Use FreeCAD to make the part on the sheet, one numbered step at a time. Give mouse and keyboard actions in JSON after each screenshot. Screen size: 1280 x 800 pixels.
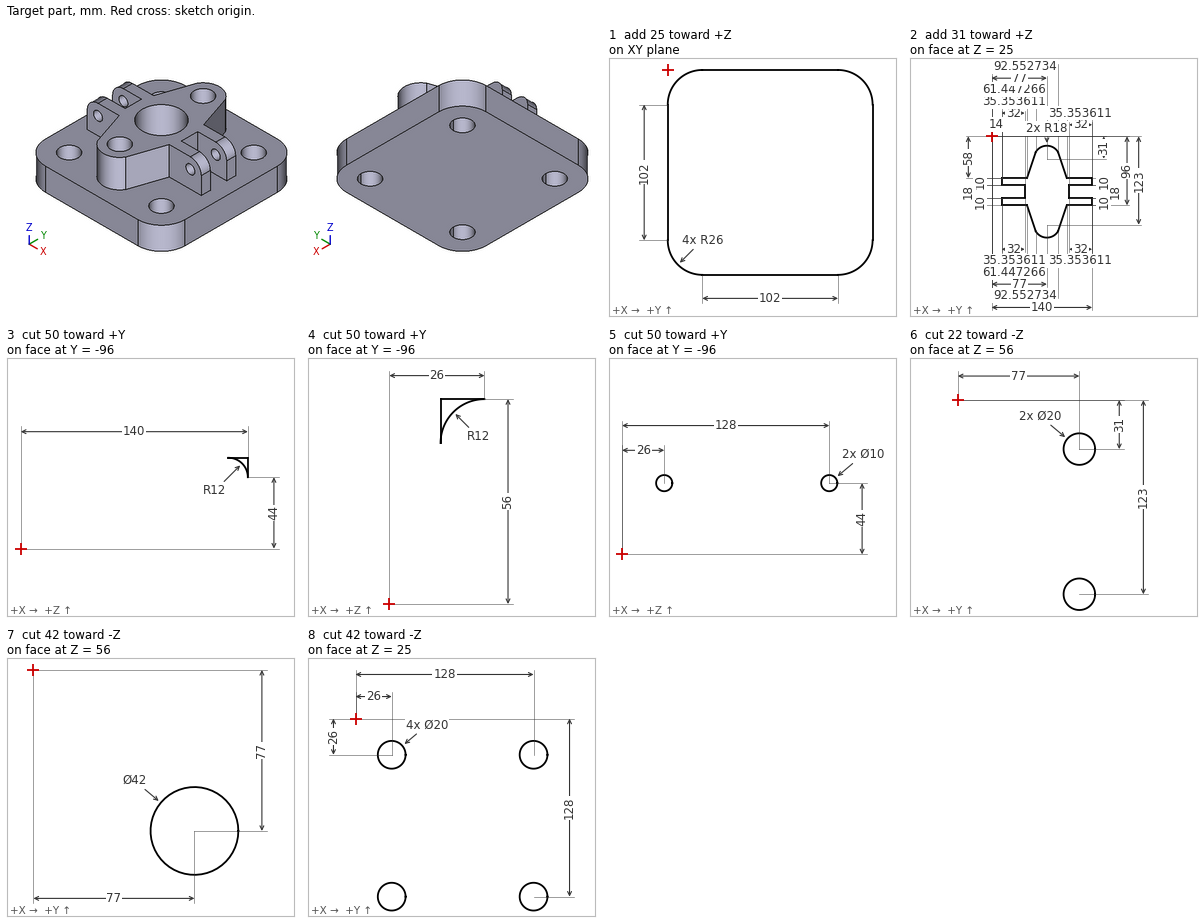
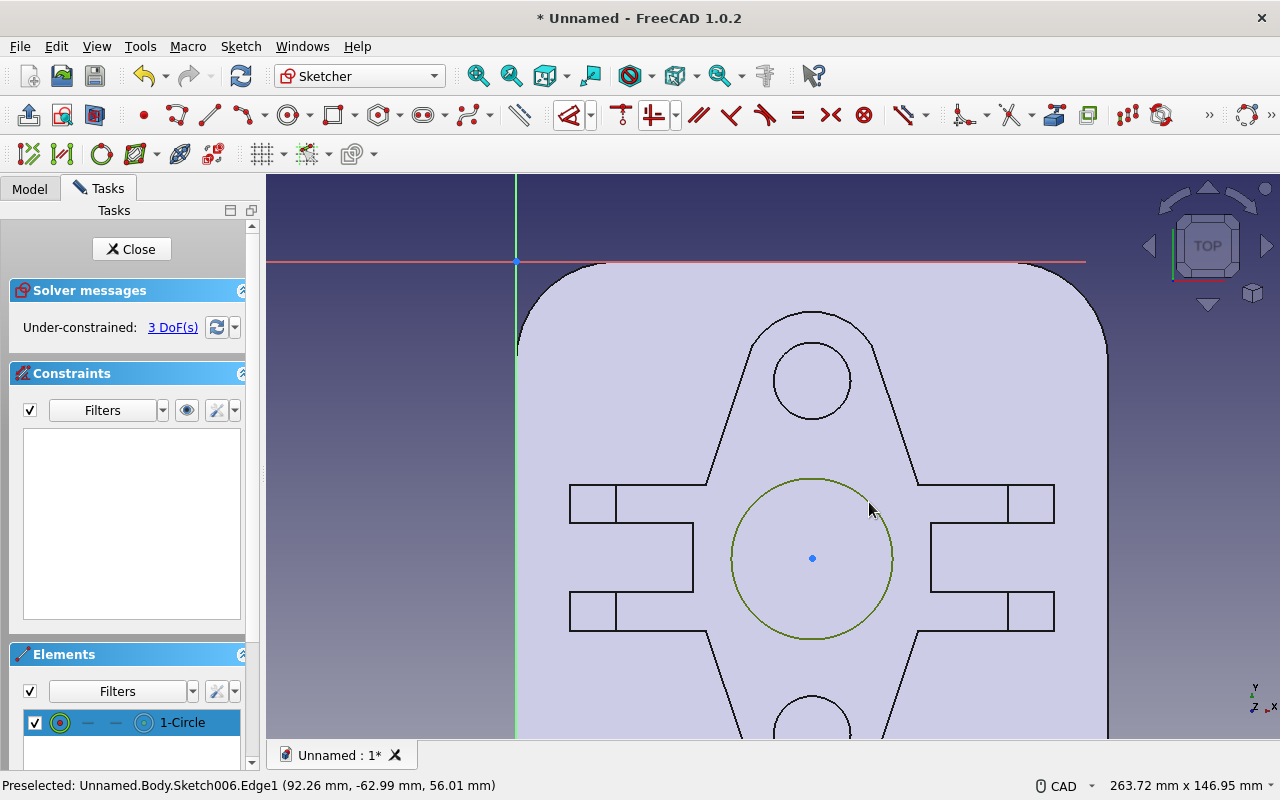
{"action": "key", "text": "k o"}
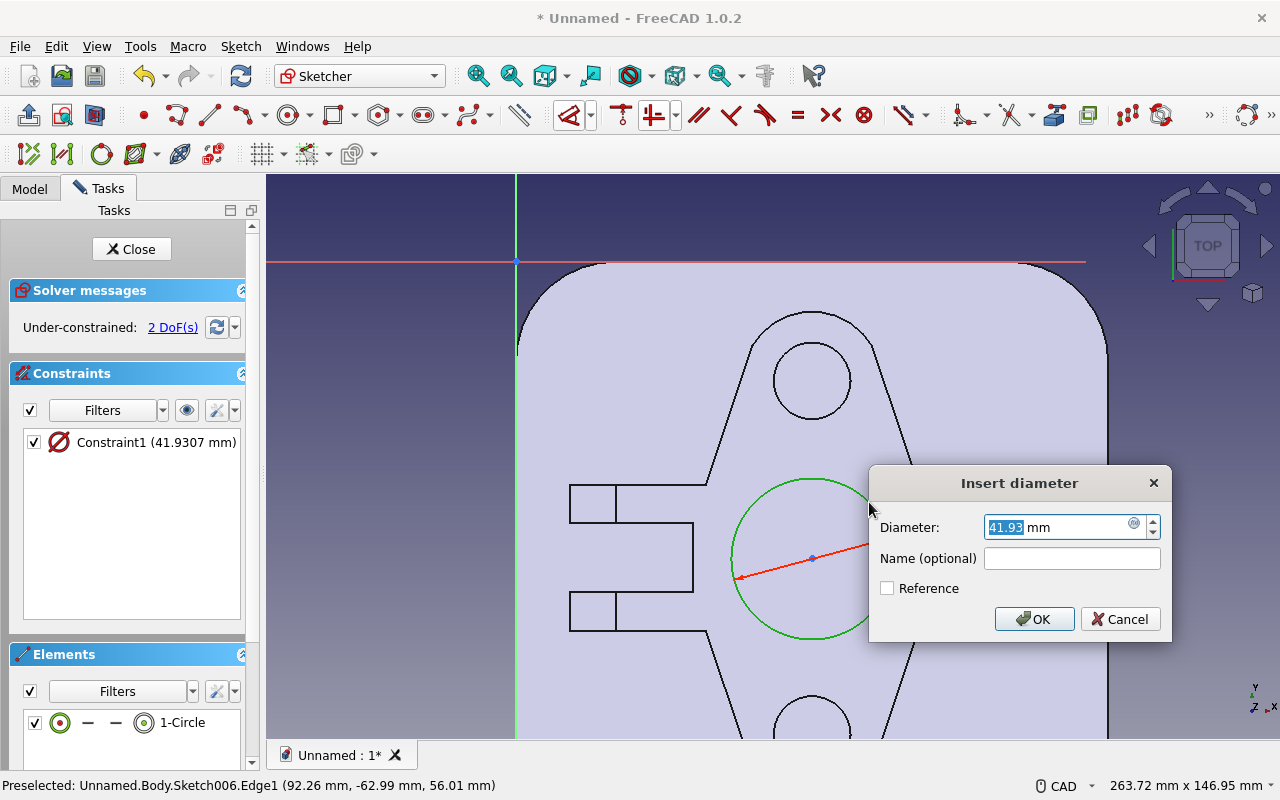
{"action": "type", "text": "42"}
{"action": "key", "text": "Return"}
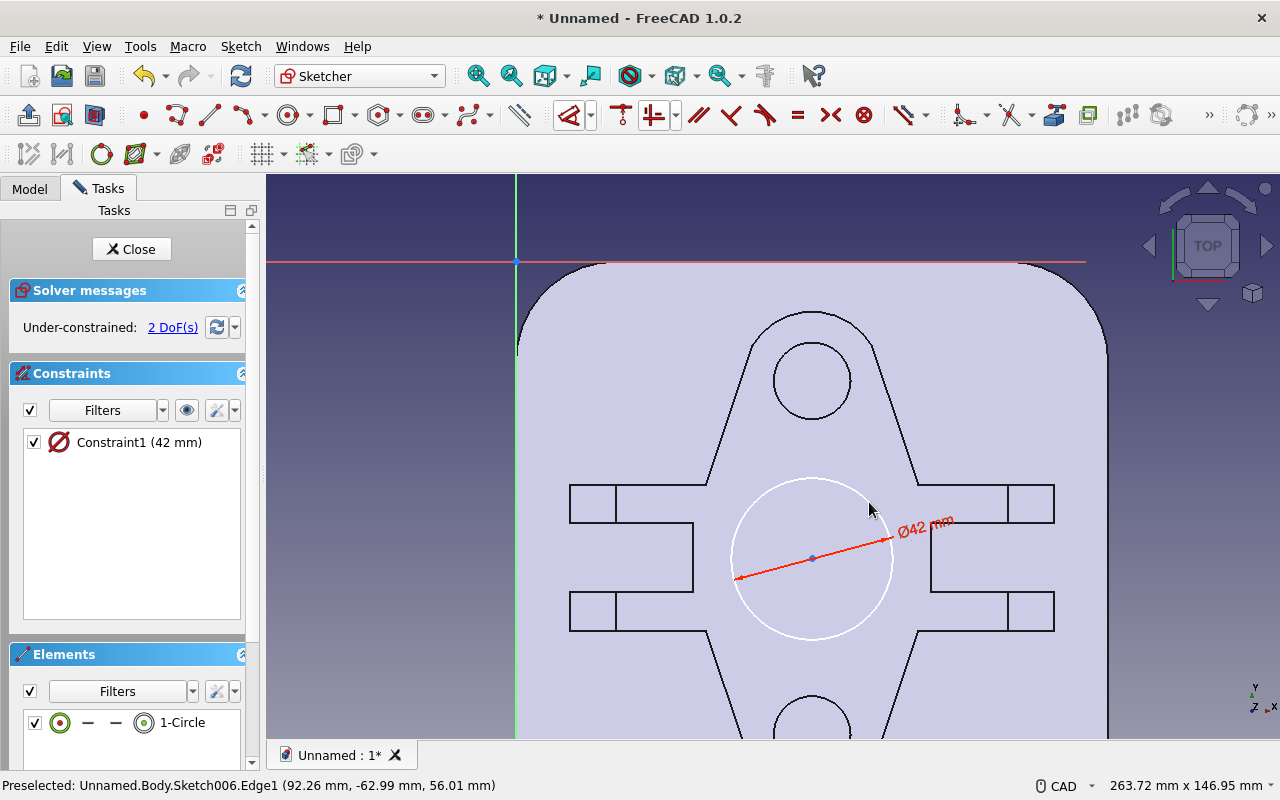
{"action": "left_click", "coordinate": [812, 559]}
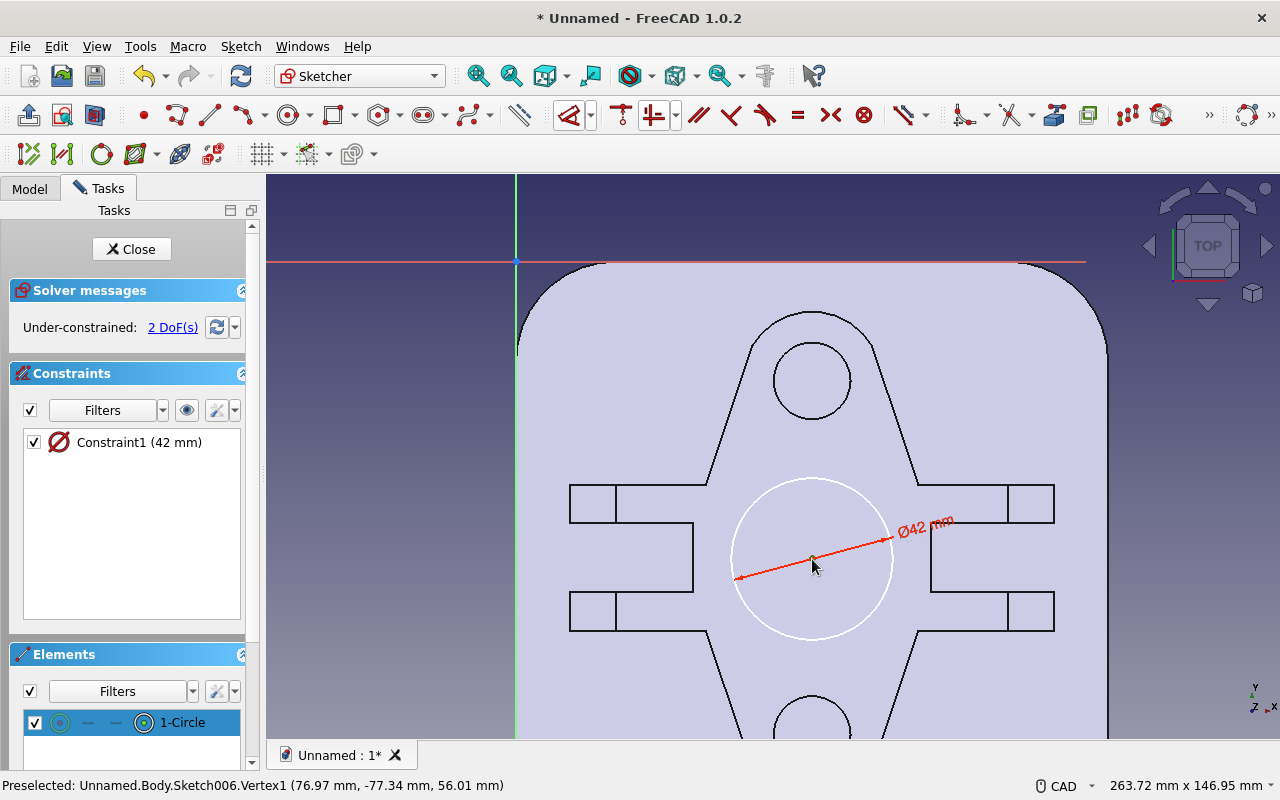
{"action": "left_click", "coordinate": [590, 116]}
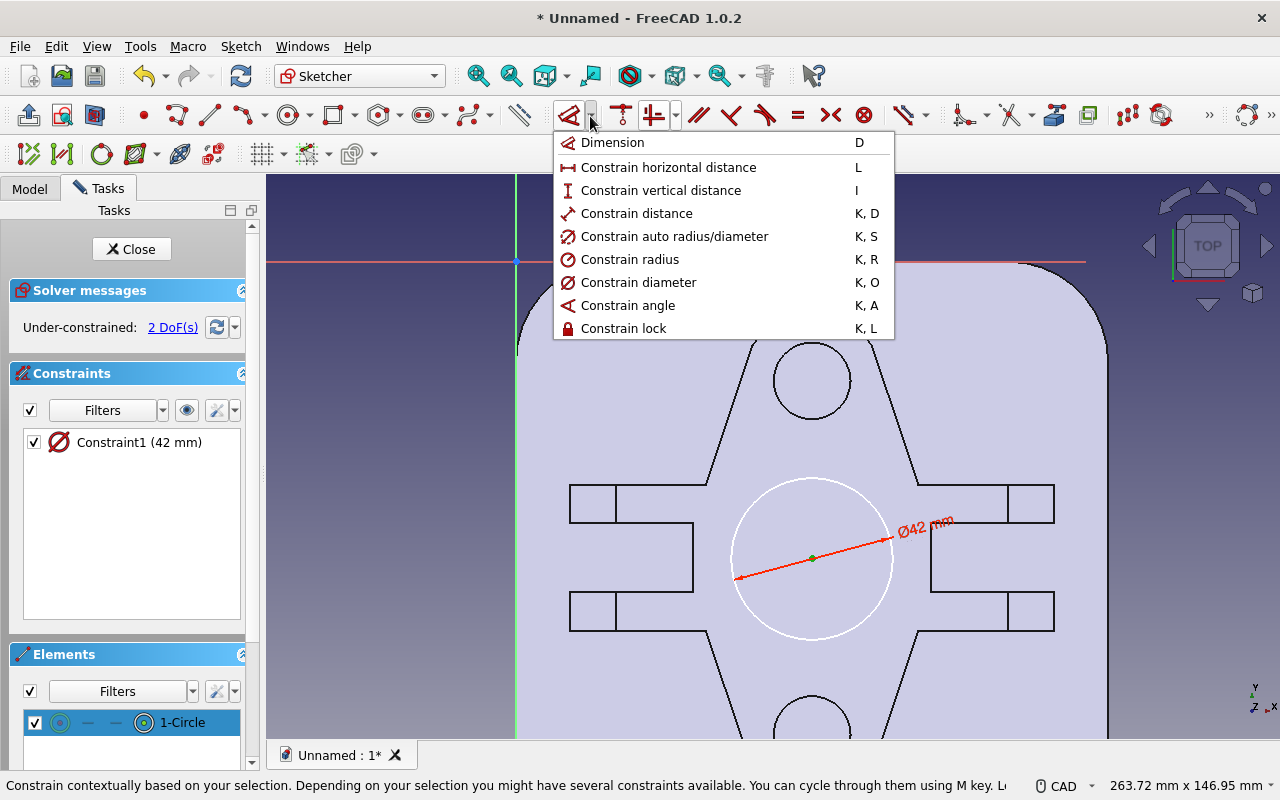
{"action": "left_click", "coordinate": [724, 168]}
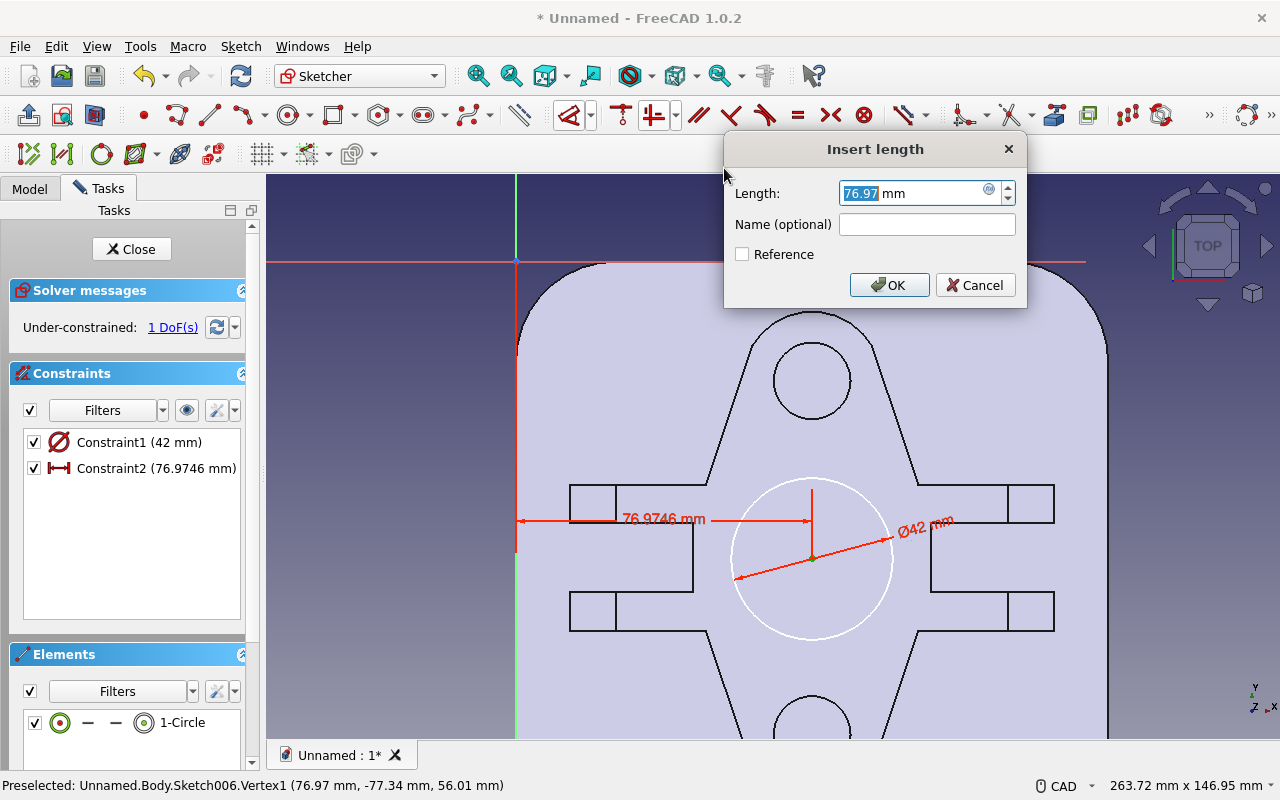
{"action": "type", "text": "77"}
{"action": "key", "text": "Return"}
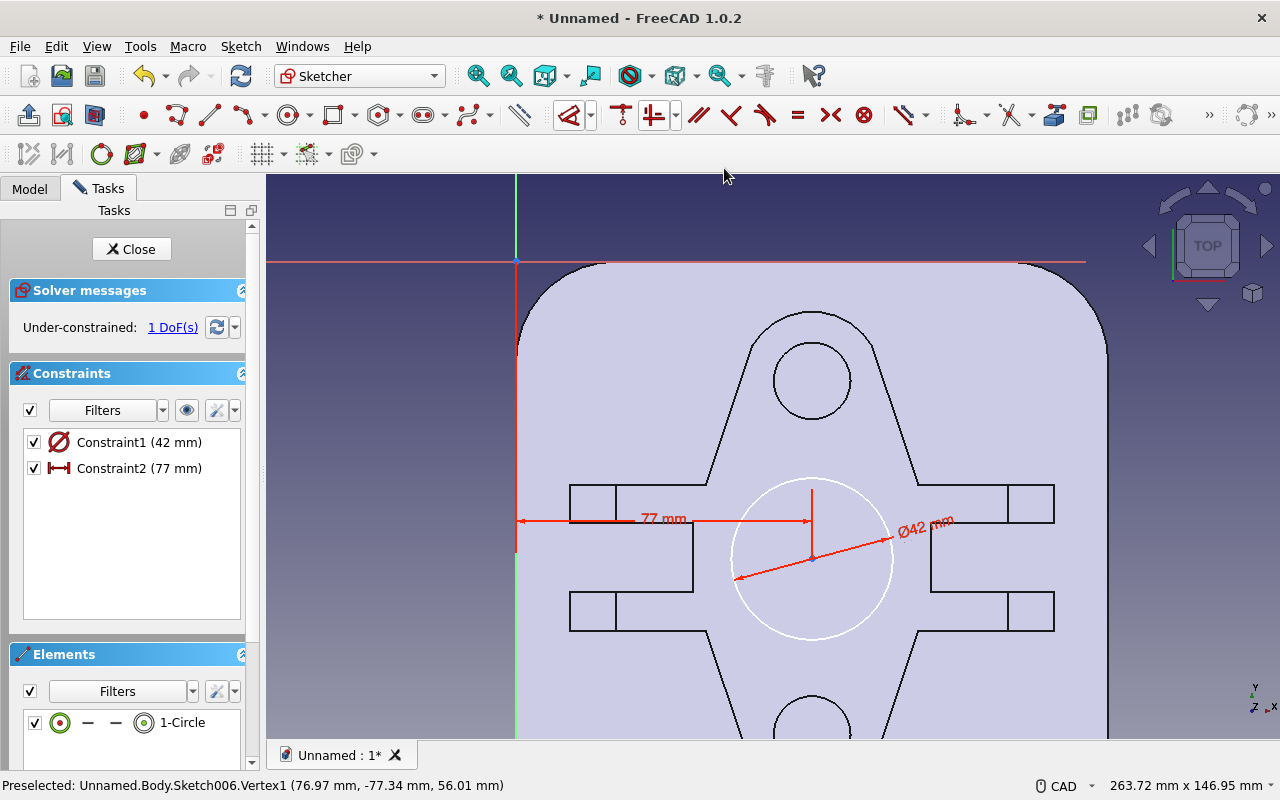
{"action": "left_click", "coordinate": [812, 559]}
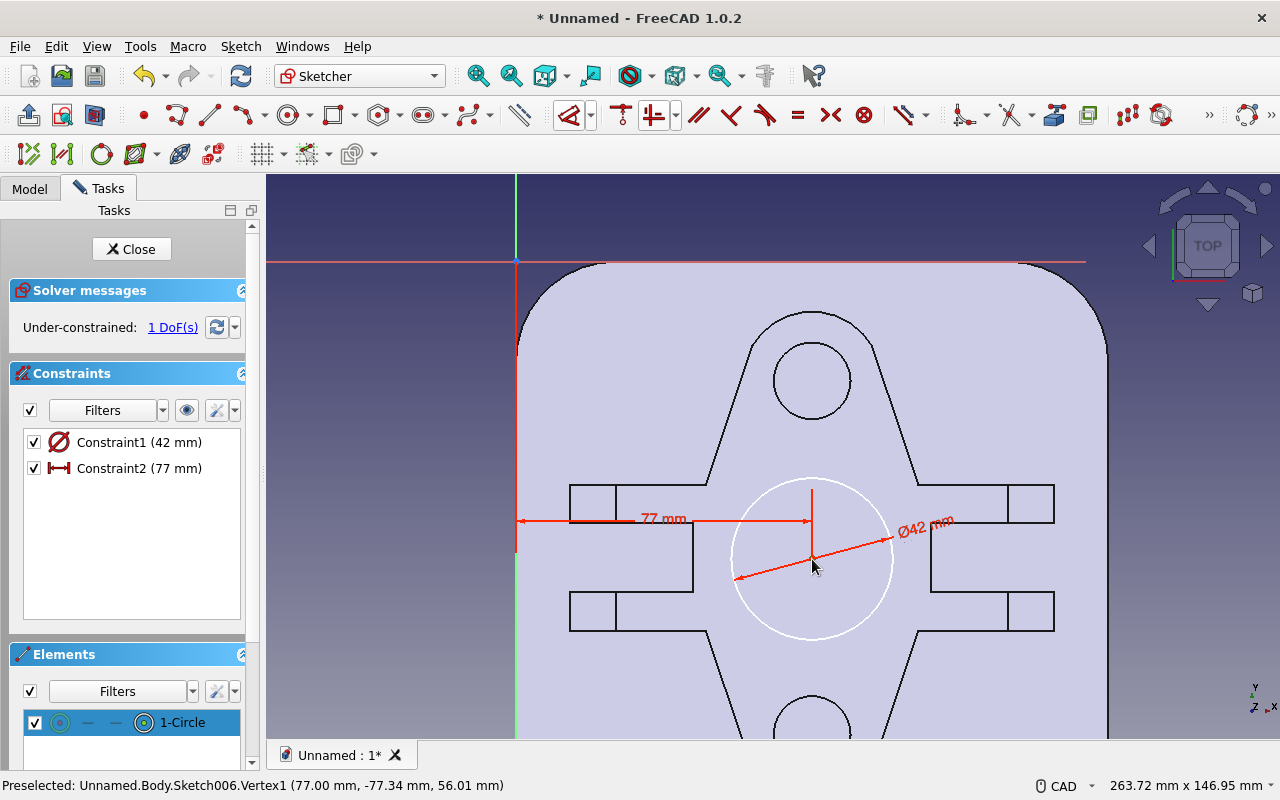
{"action": "left_click", "coordinate": [590, 116]}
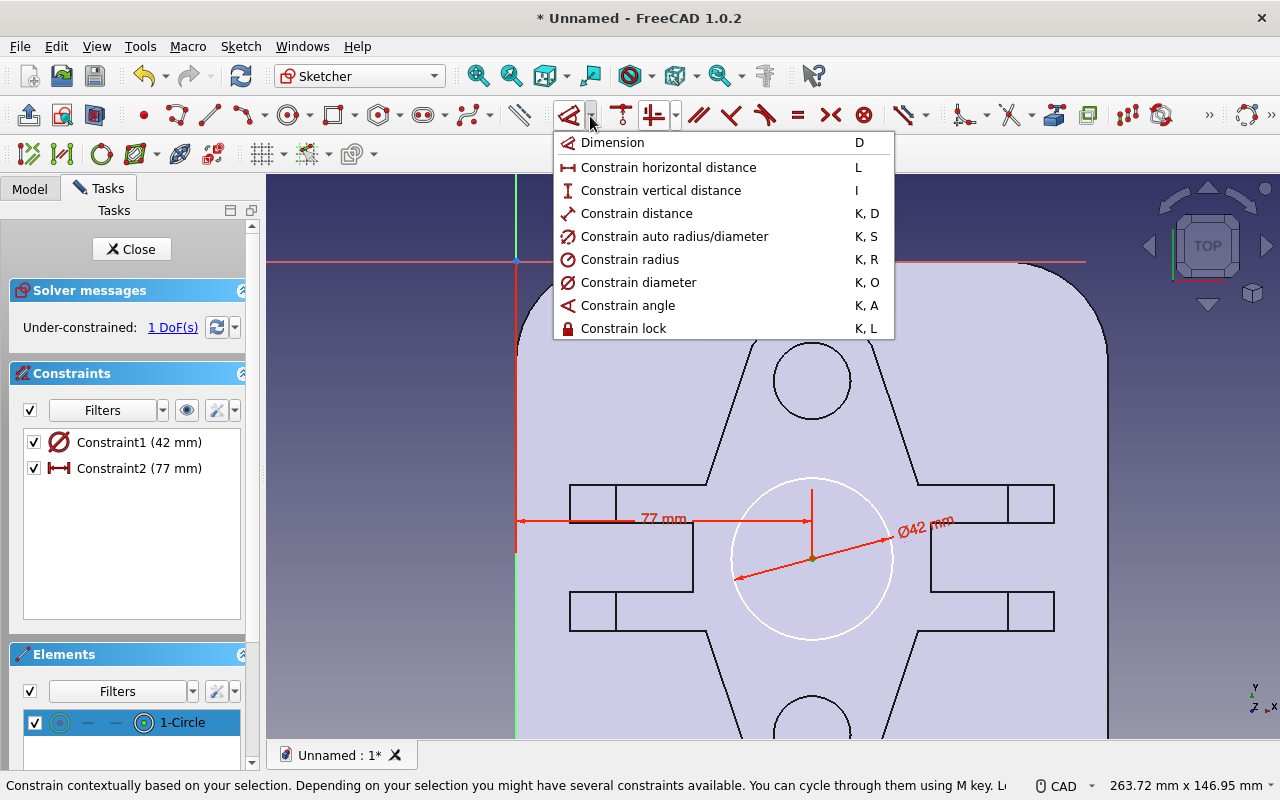
{"action": "left_click", "coordinate": [724, 190]}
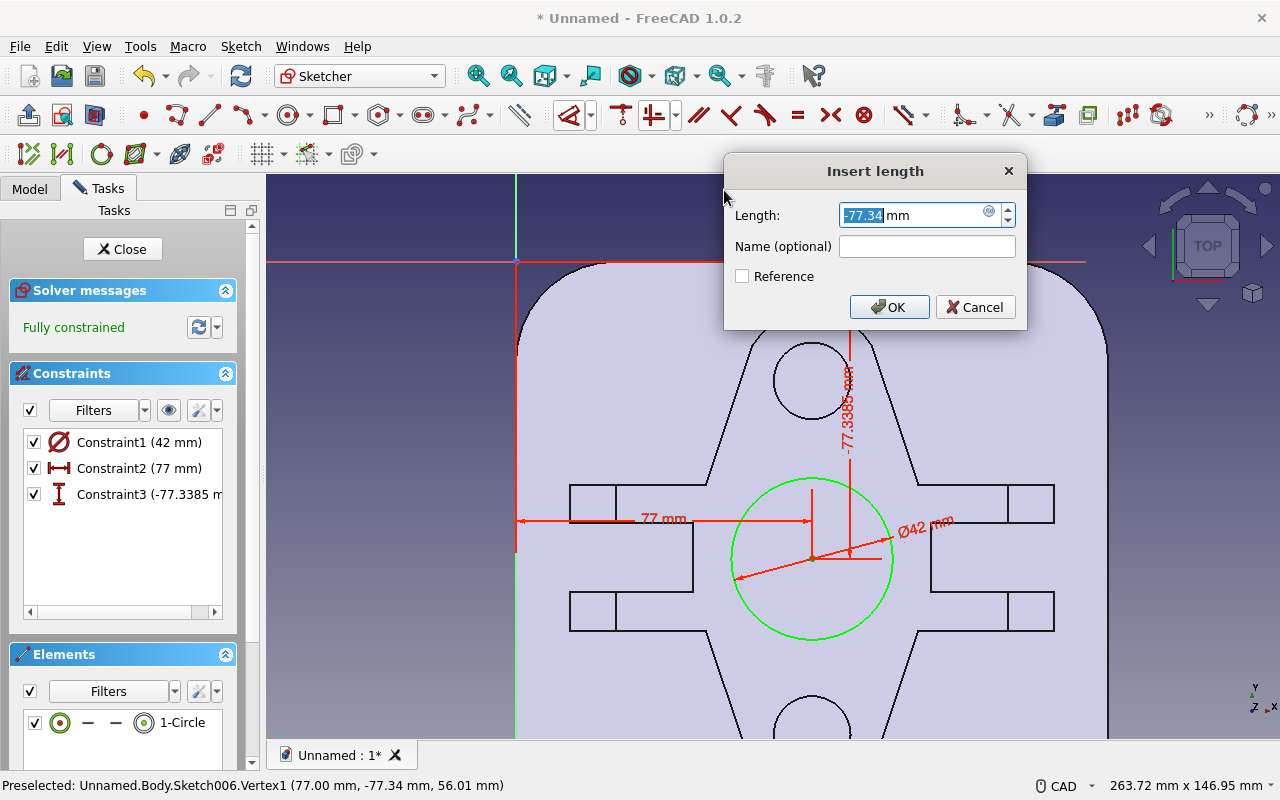
{"action": "type", "text": "-77"}
{"action": "key", "text": "Return"}